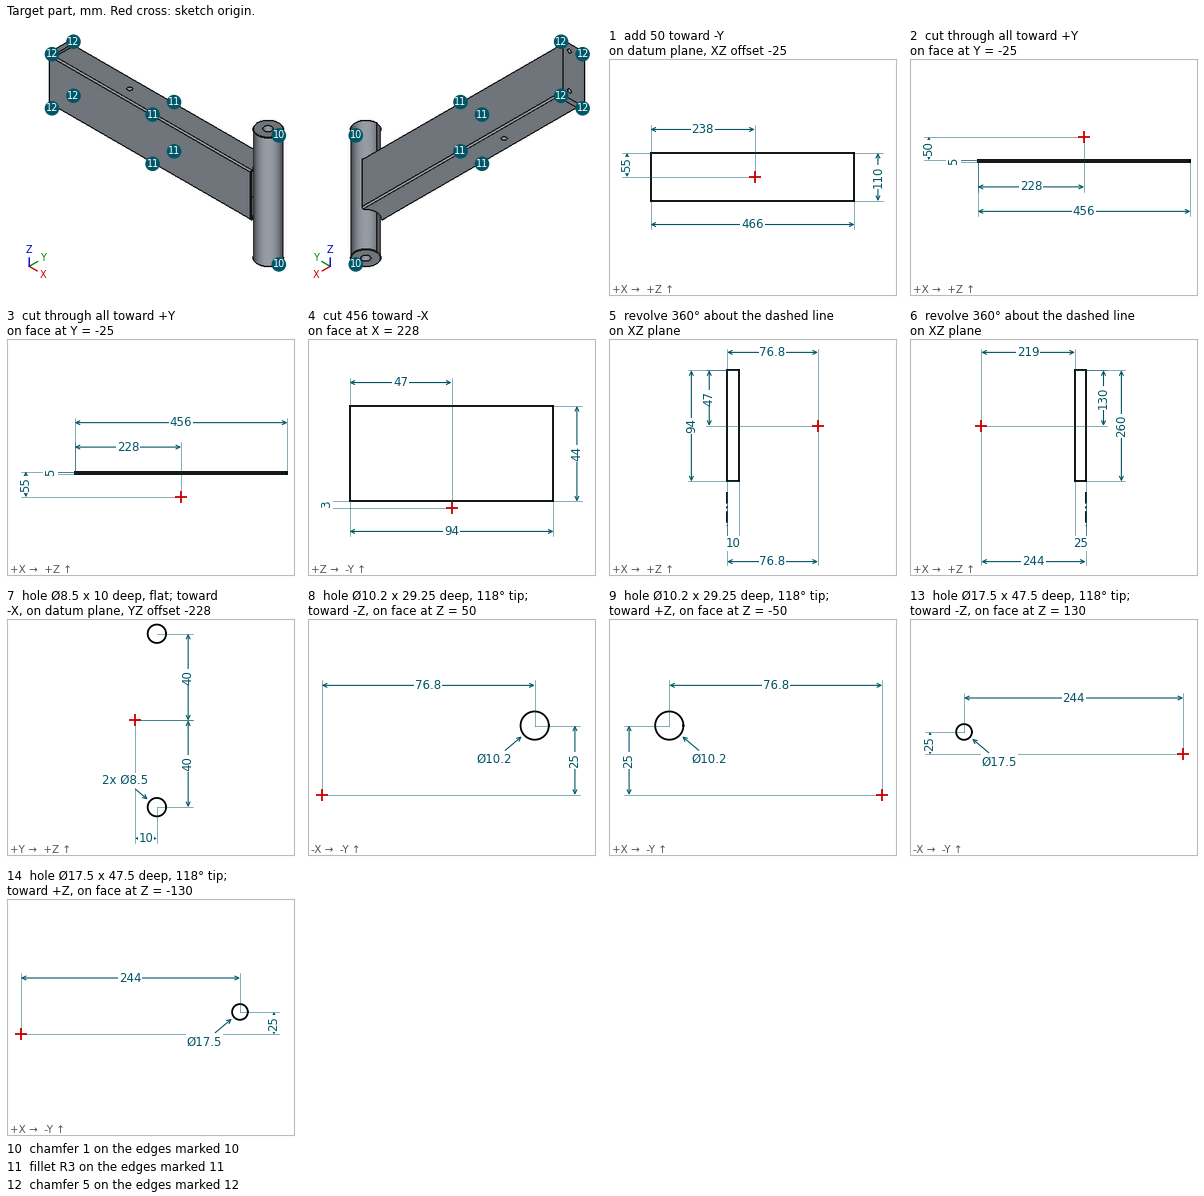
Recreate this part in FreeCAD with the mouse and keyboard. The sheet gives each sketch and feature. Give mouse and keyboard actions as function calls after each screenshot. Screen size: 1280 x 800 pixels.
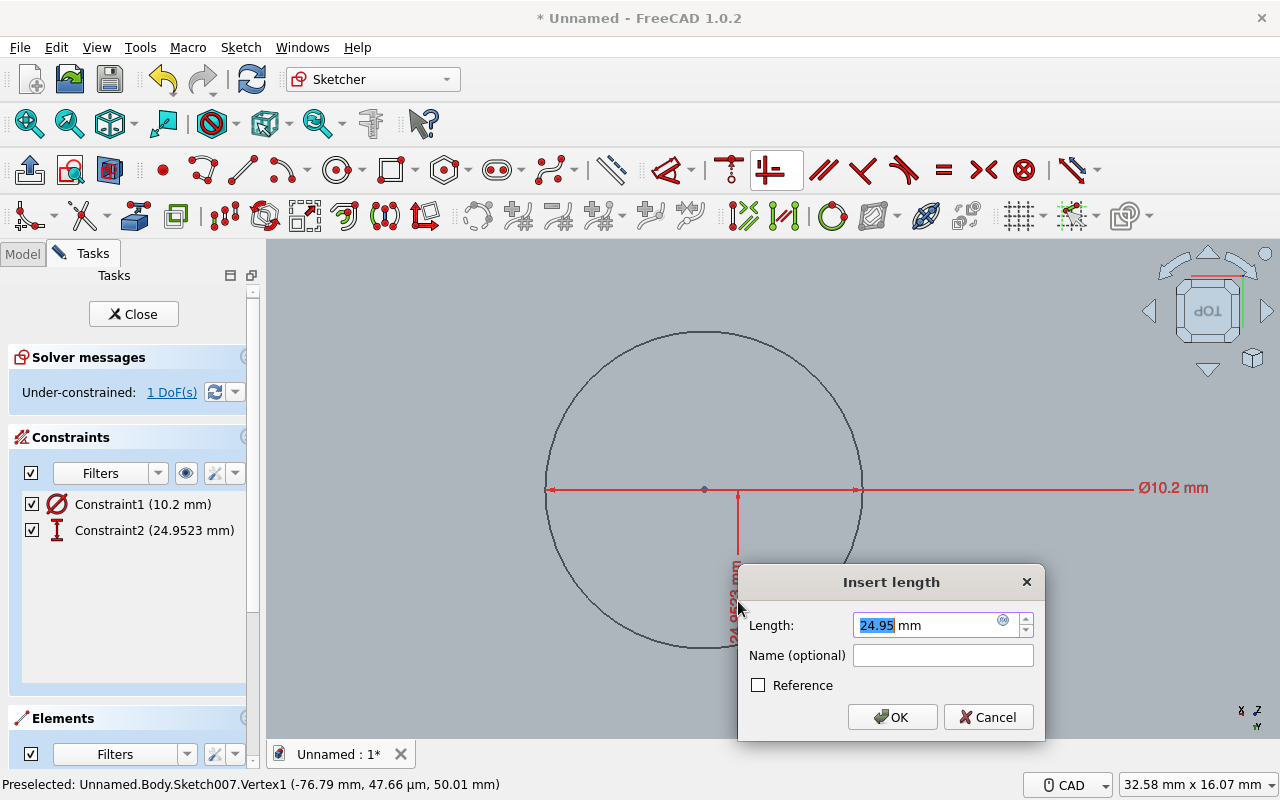
text(25)
key(Return)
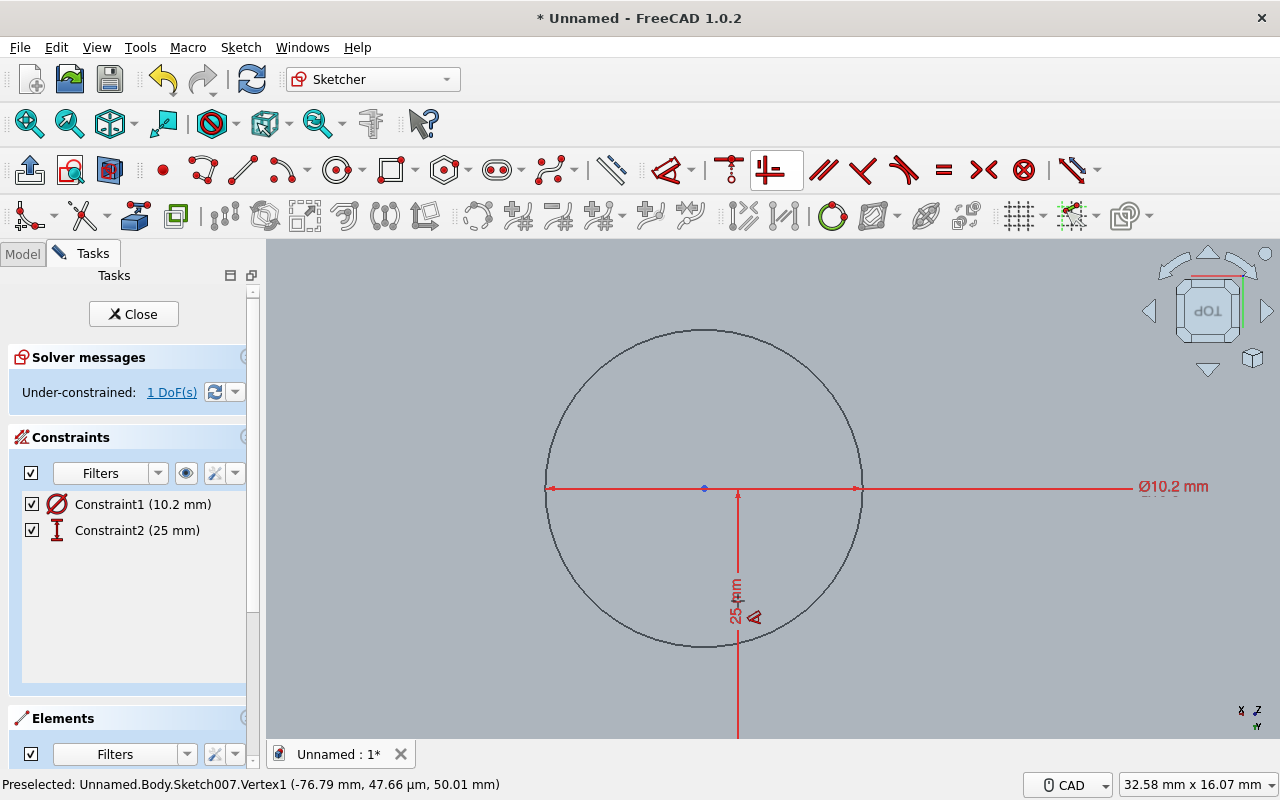
click(704, 489)
click(499, 455)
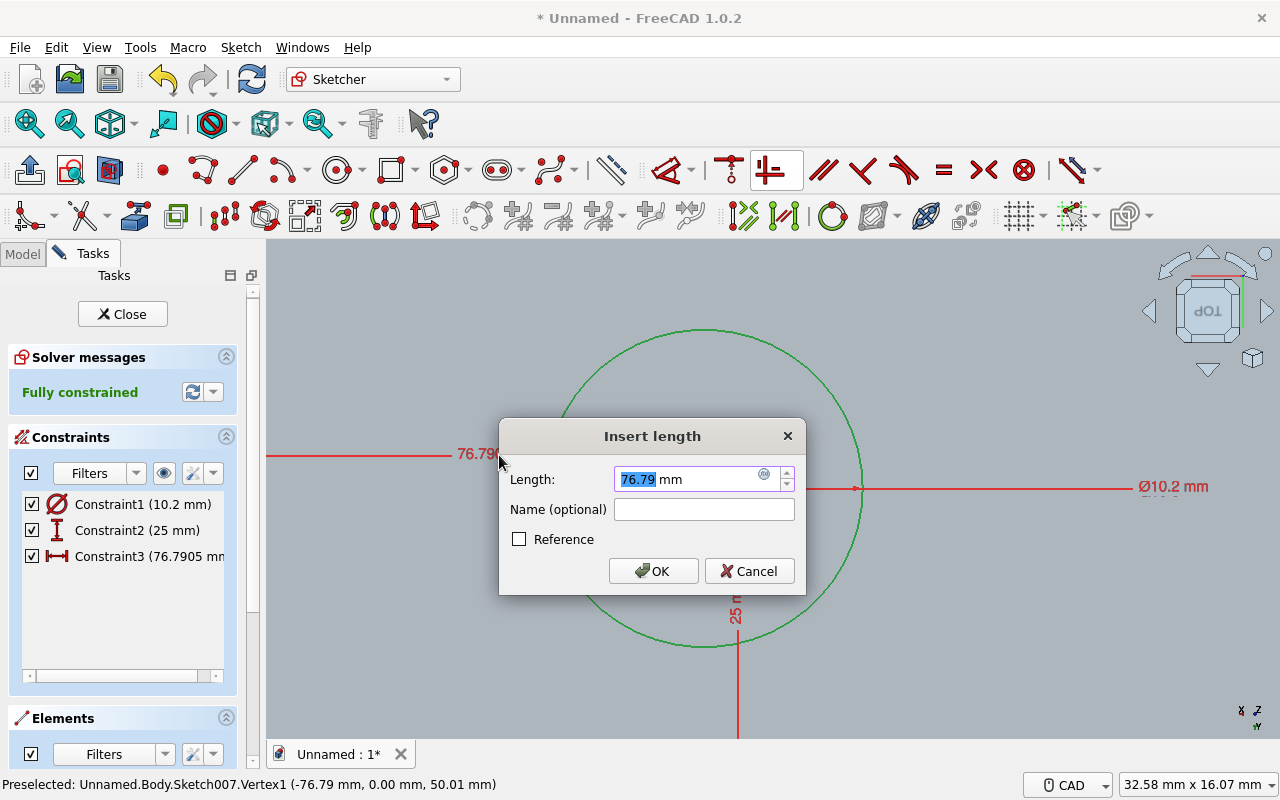
text(76.8)
key(Return)
key(Escape)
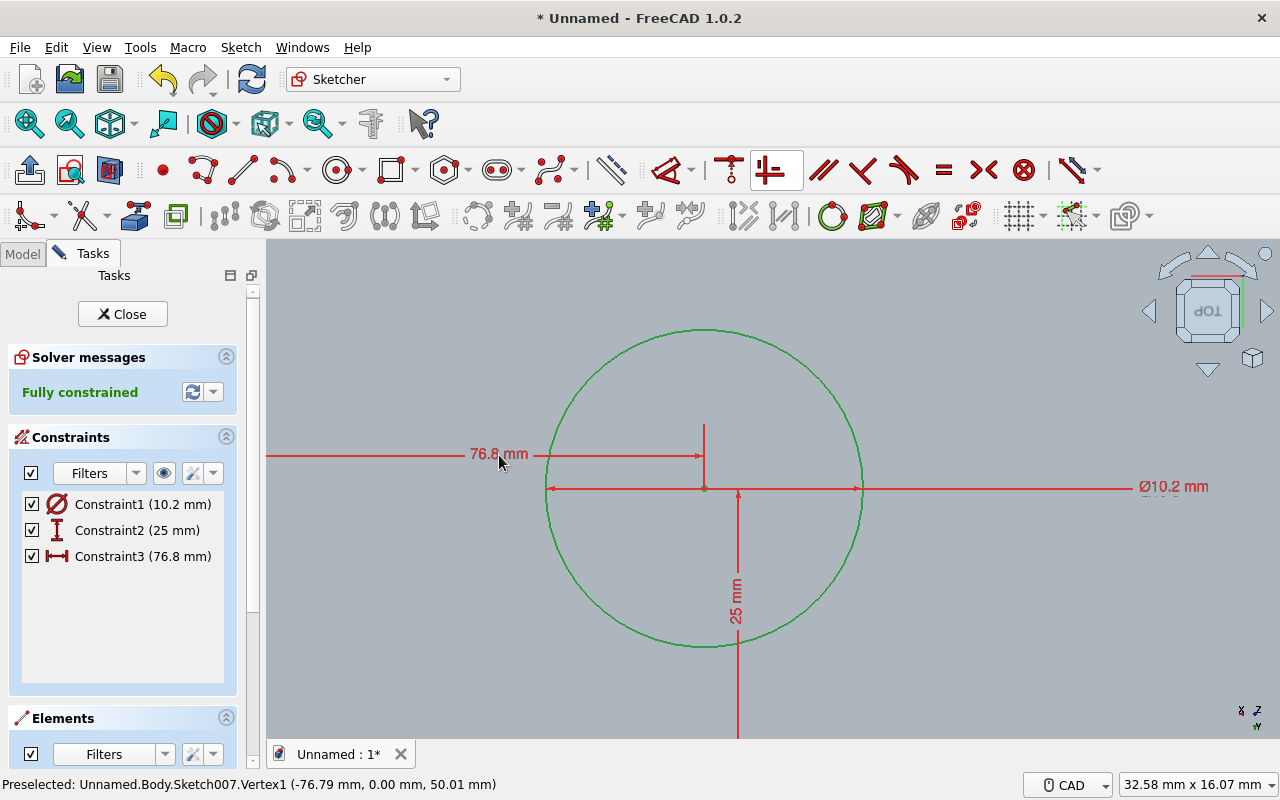
click(123, 314)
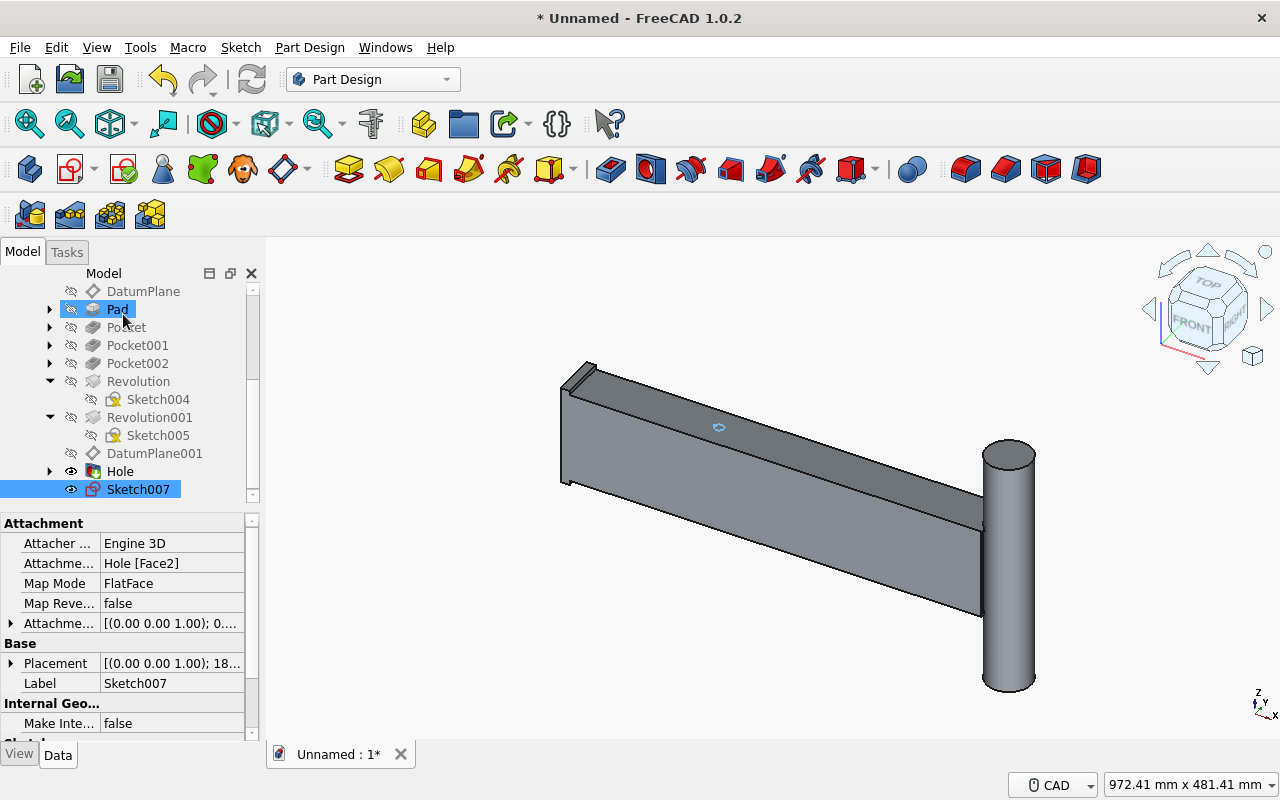
click(652, 170)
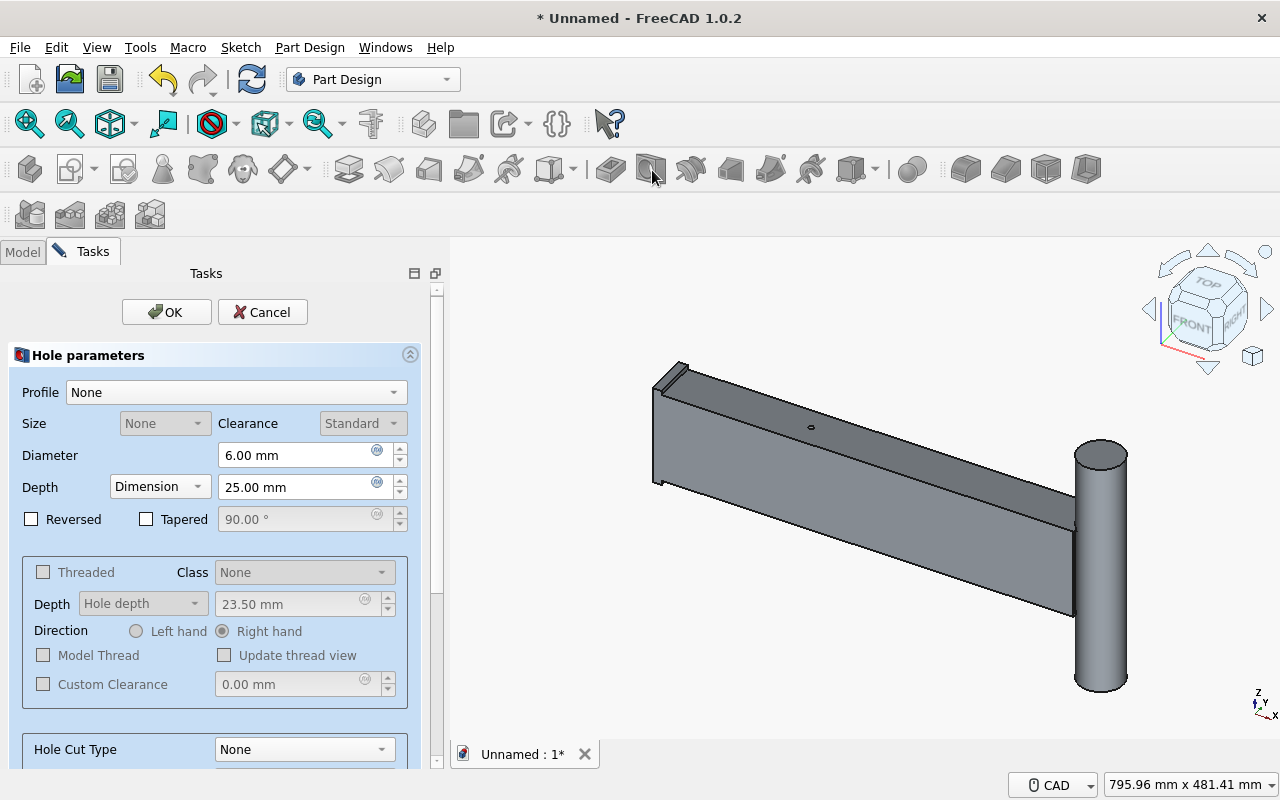
triple_click(305, 455)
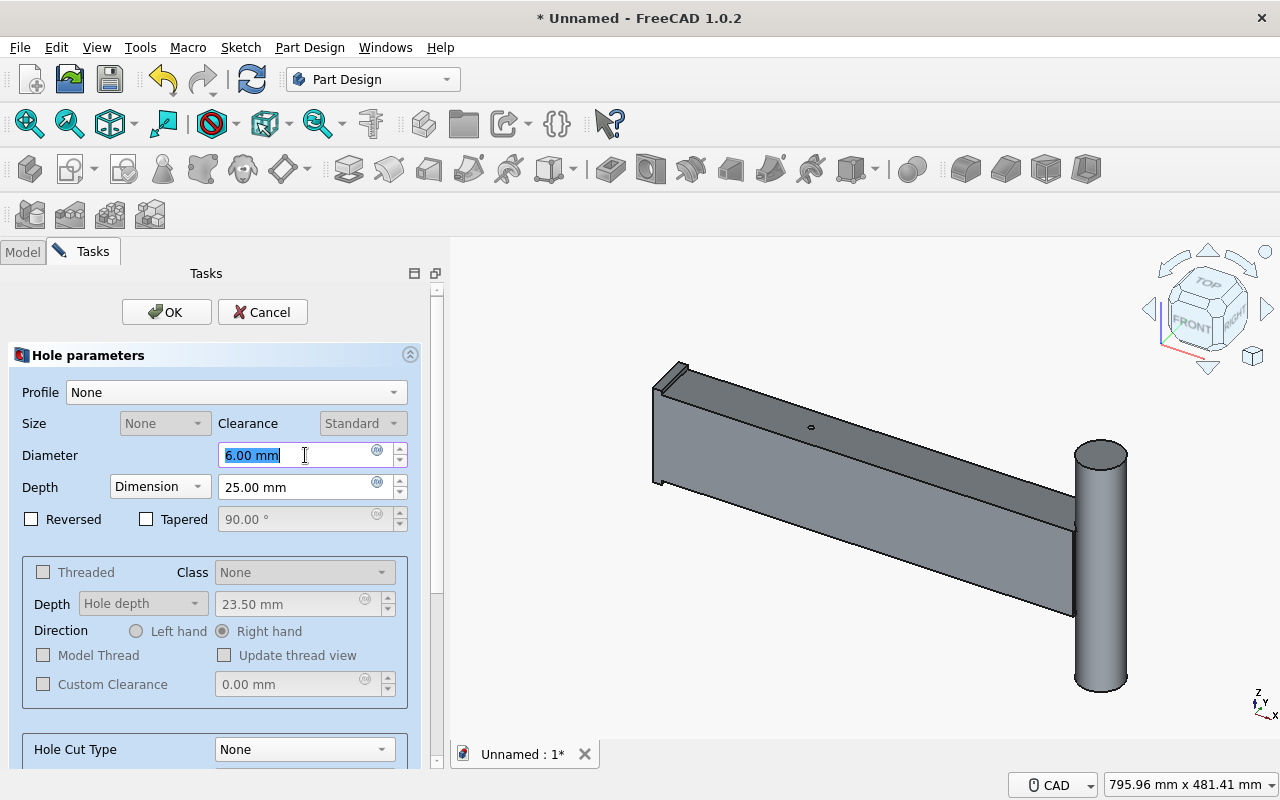
text(10.2)
key(Tab)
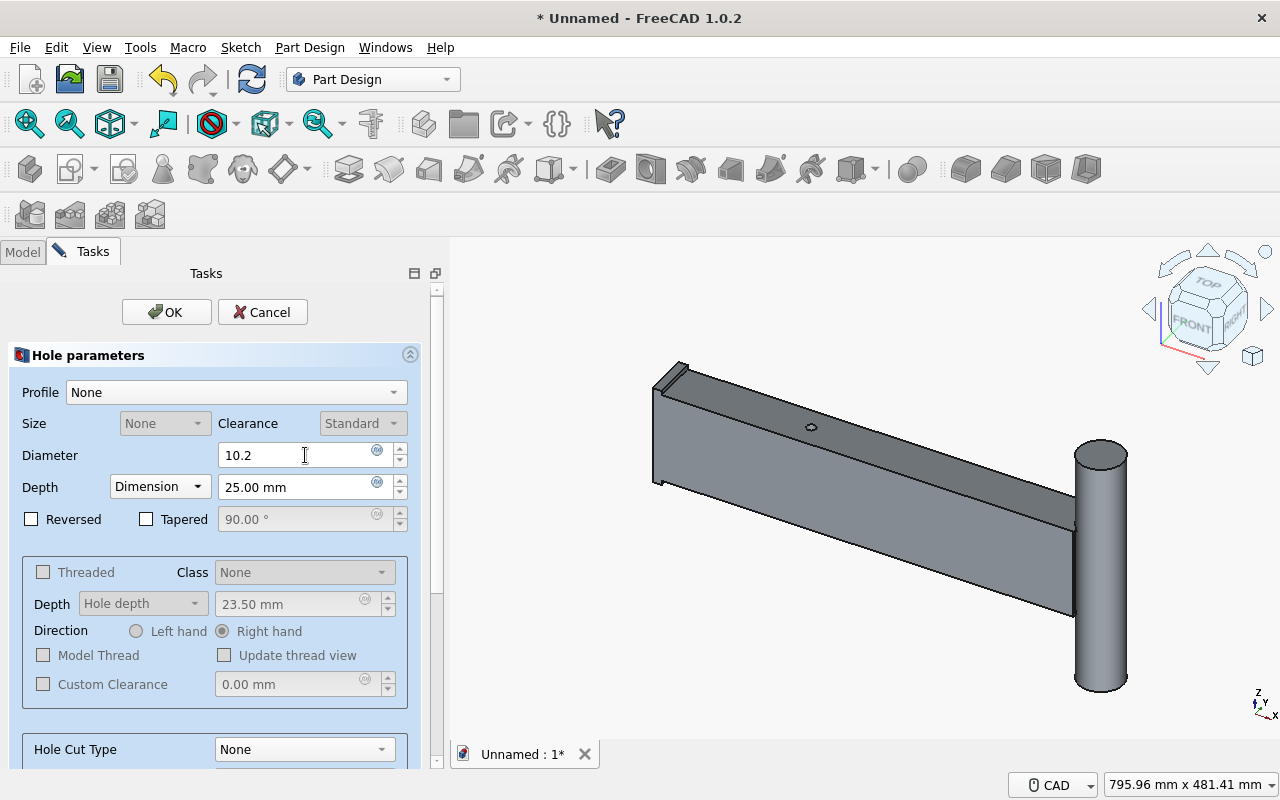
triple_click(305, 487)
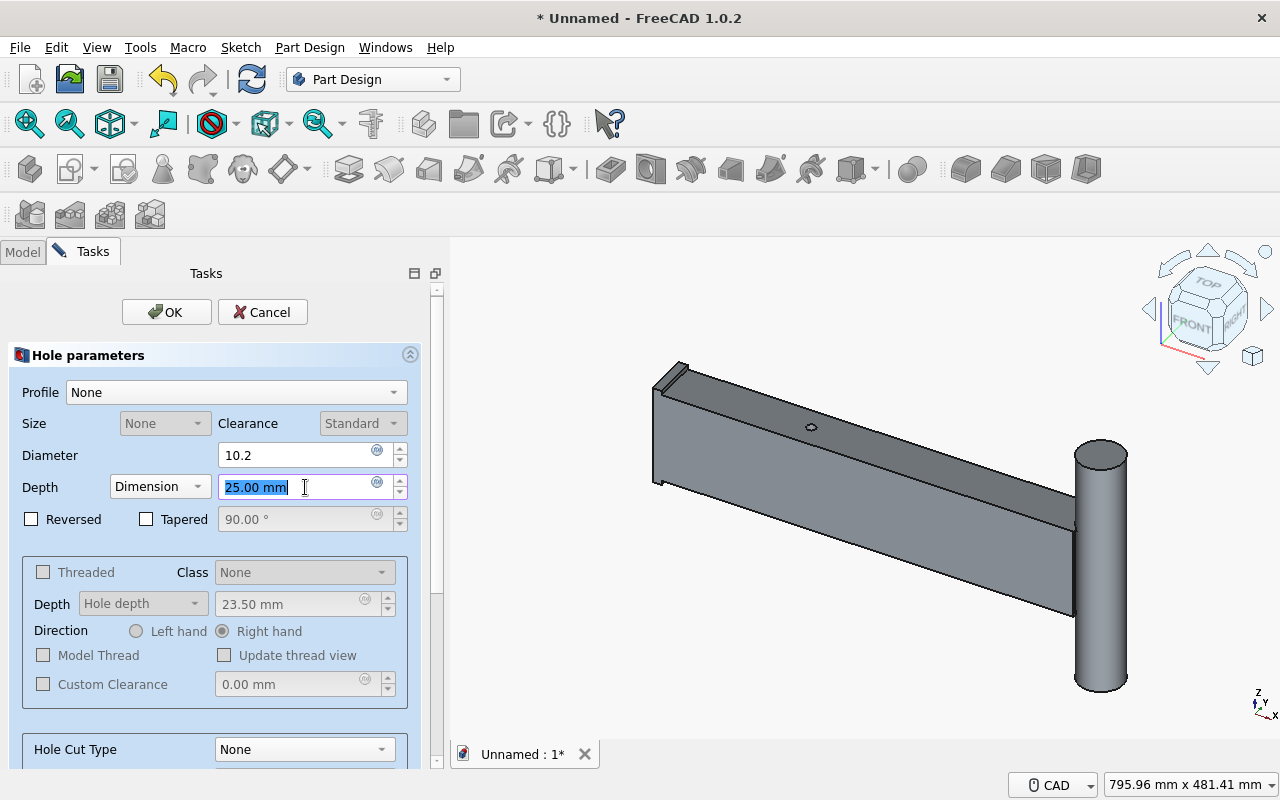
text(29.25)
key(Tab)